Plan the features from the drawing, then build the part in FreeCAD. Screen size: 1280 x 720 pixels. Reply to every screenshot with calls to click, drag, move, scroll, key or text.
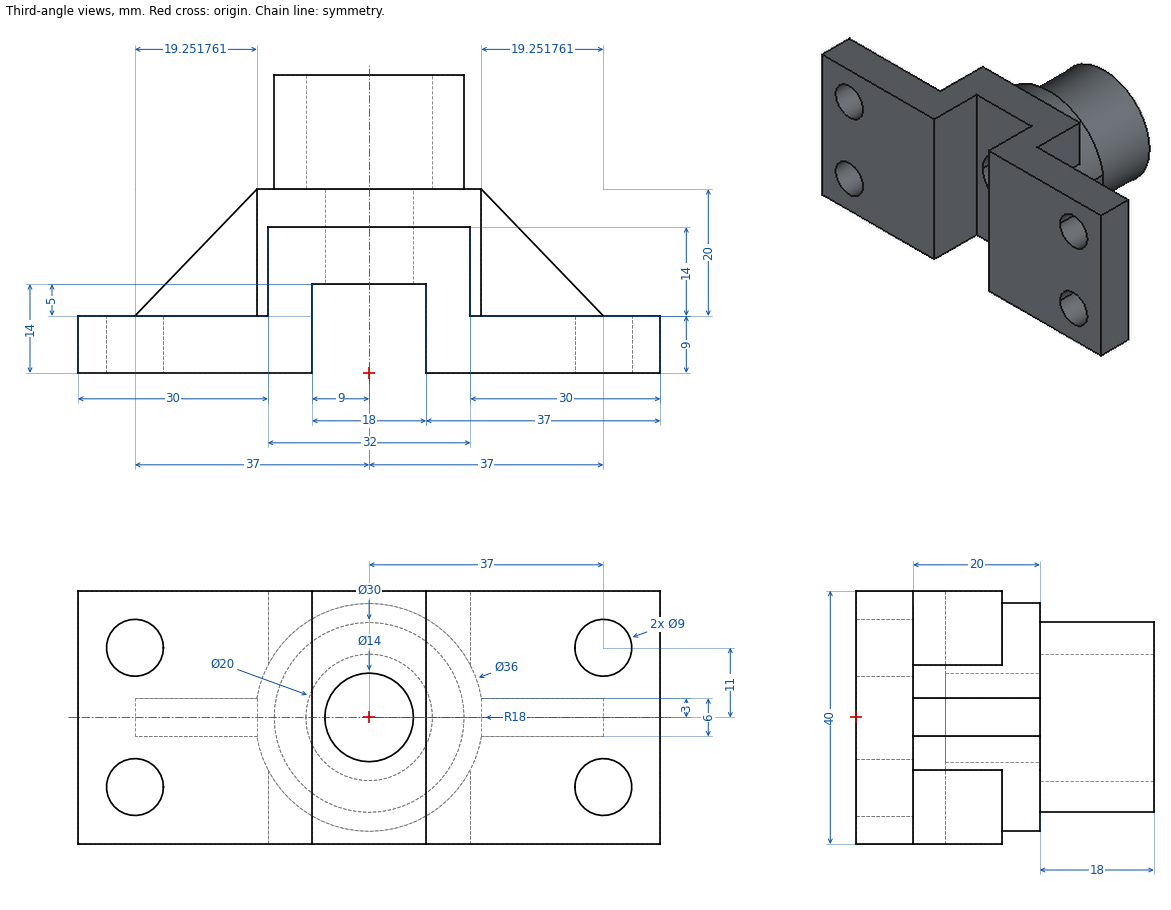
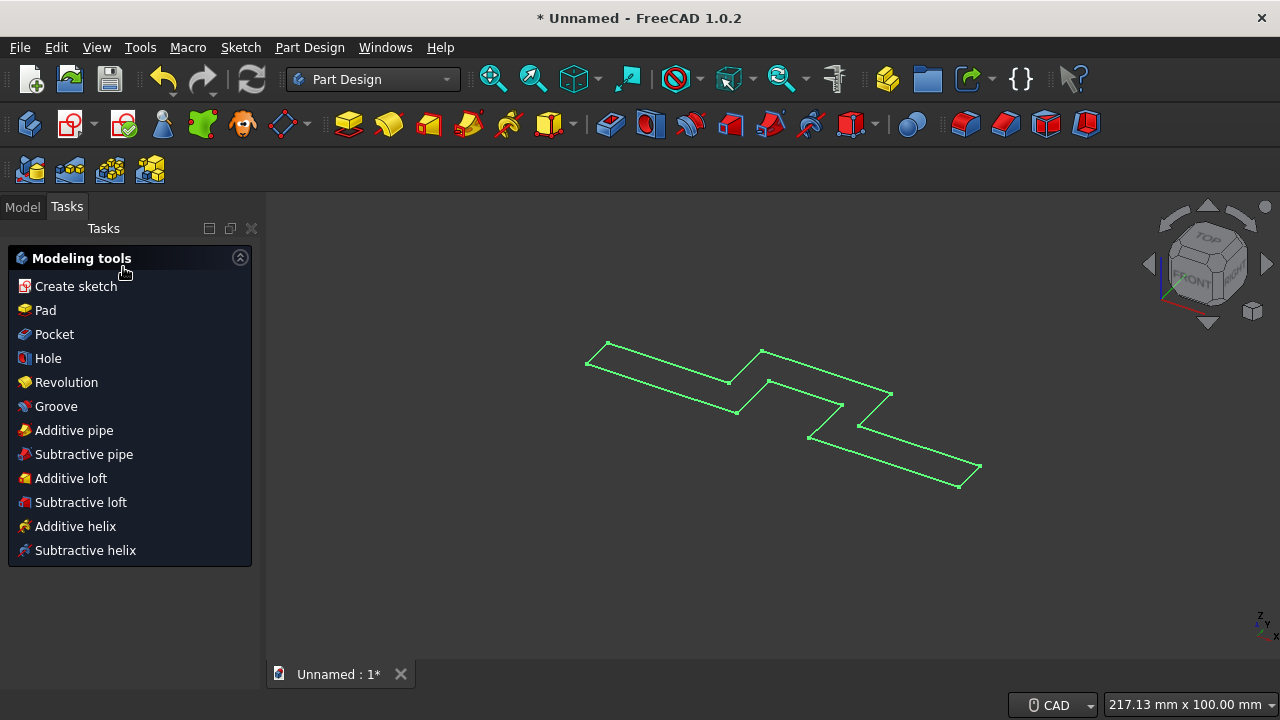
click(350, 124)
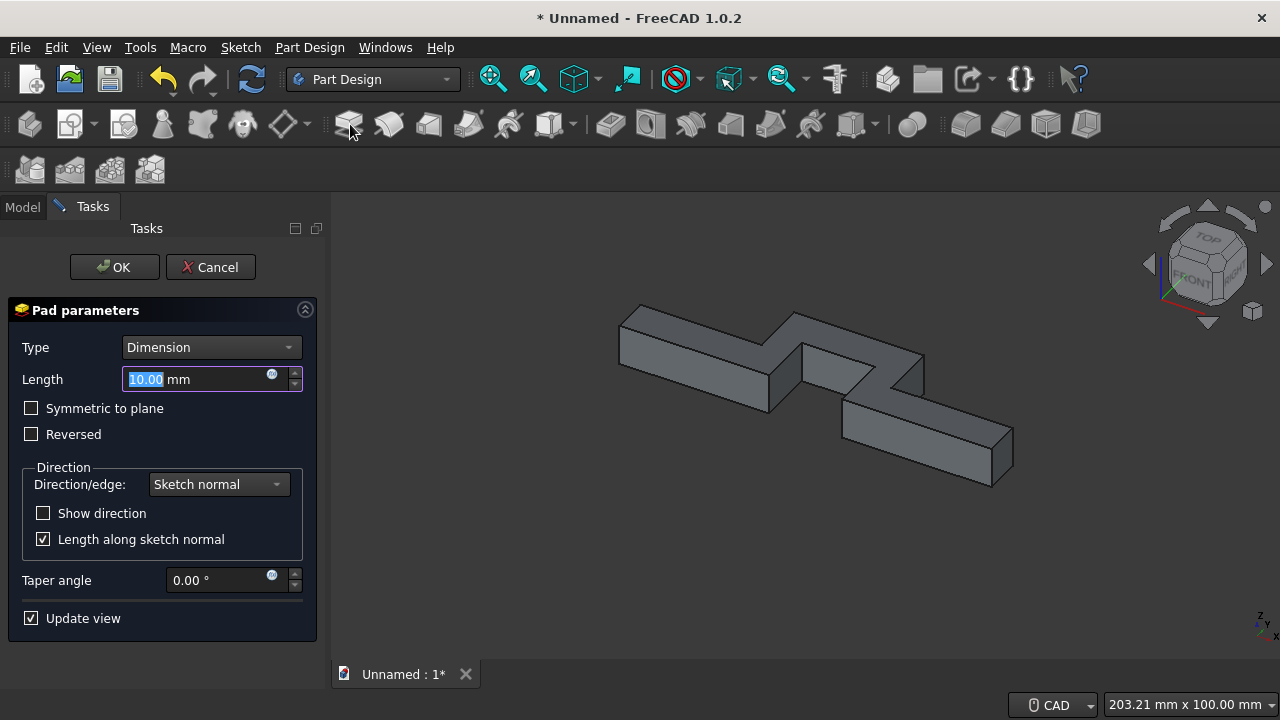
text(40)
key(Tab)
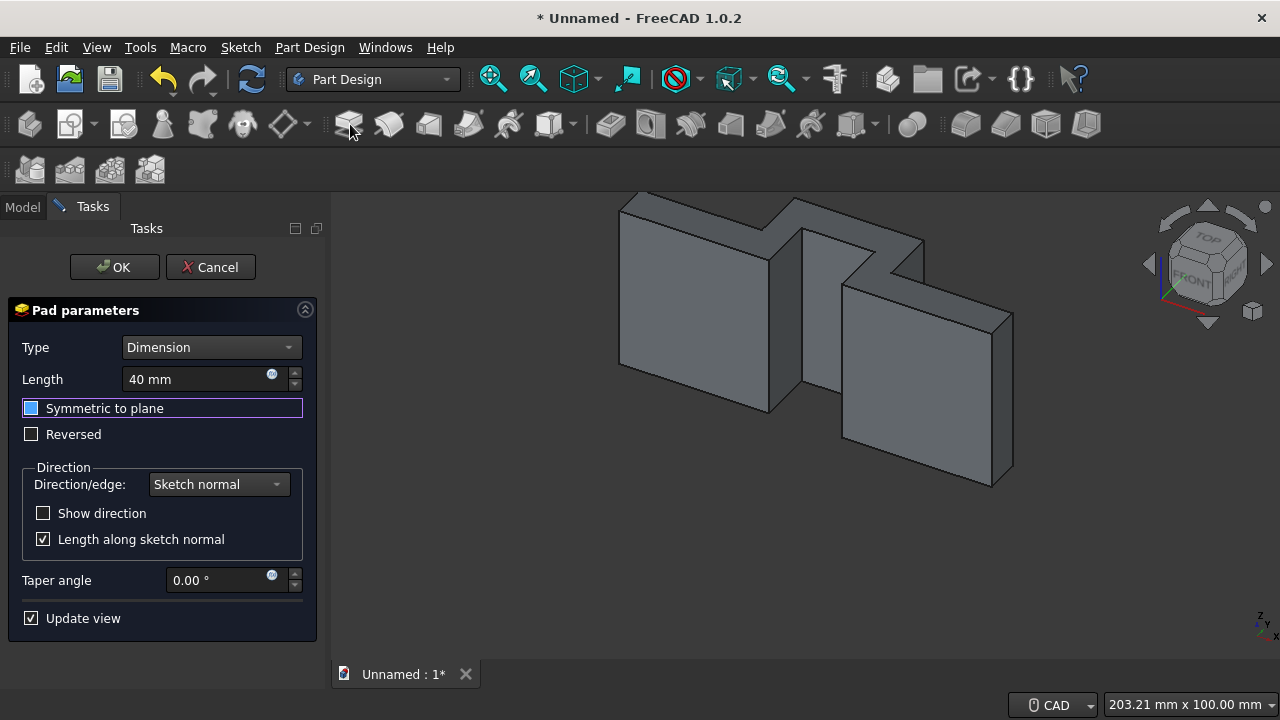
click(30, 408)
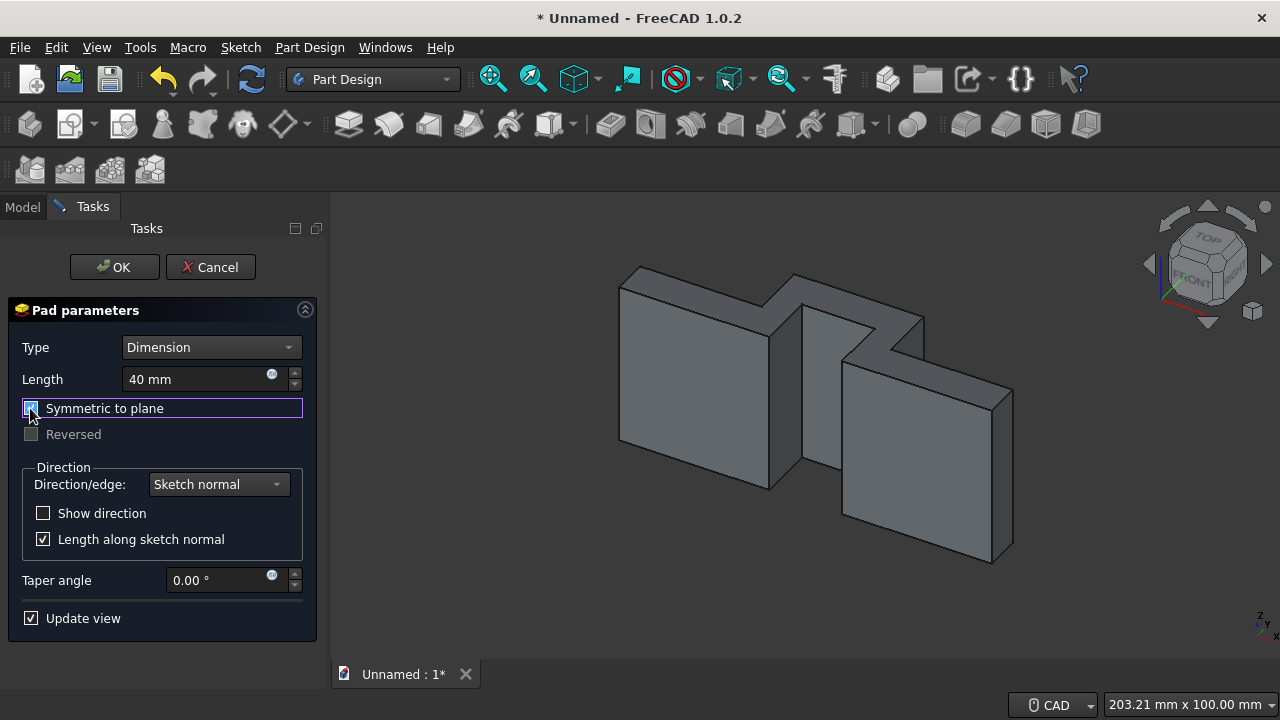
click(115, 267)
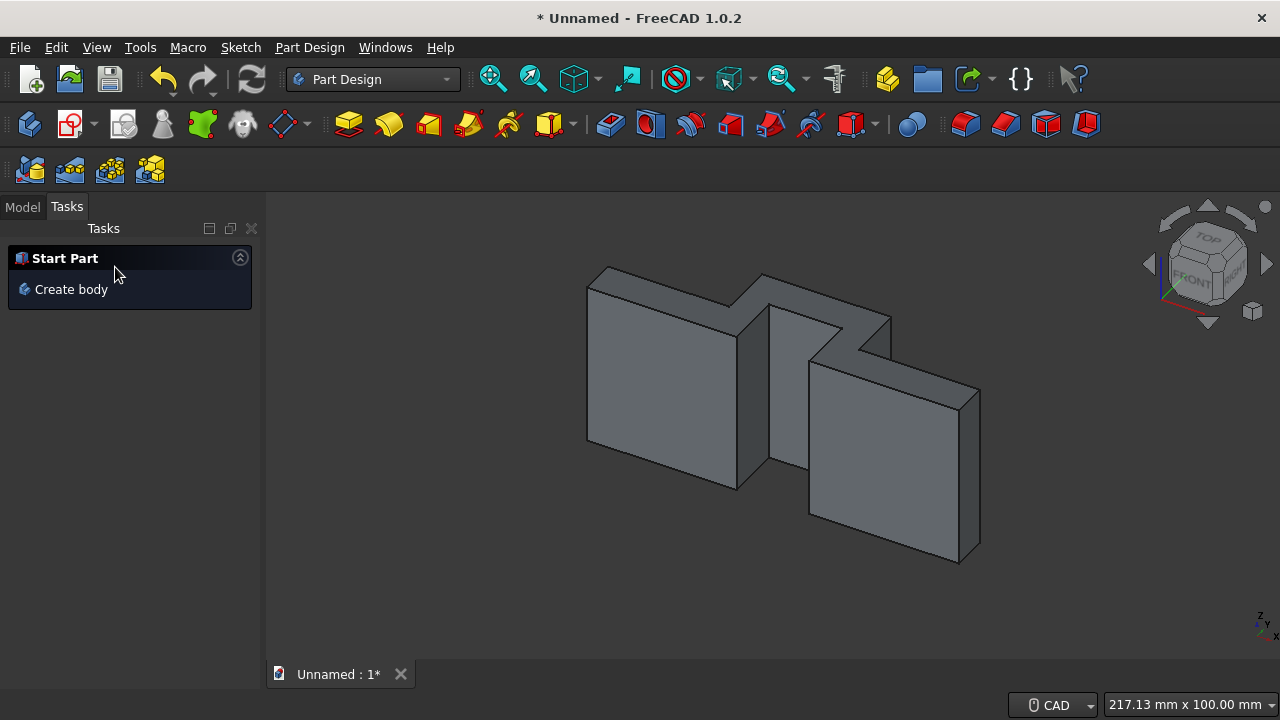
key(4)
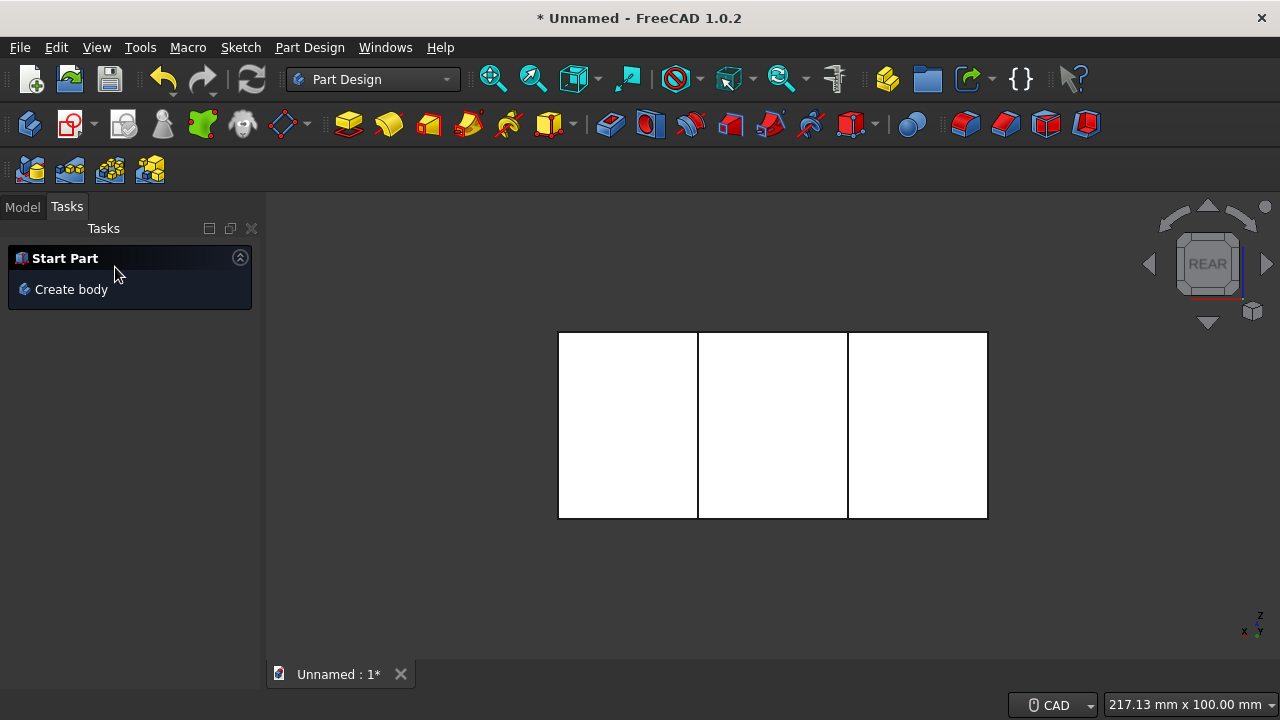
key(v)
key(f)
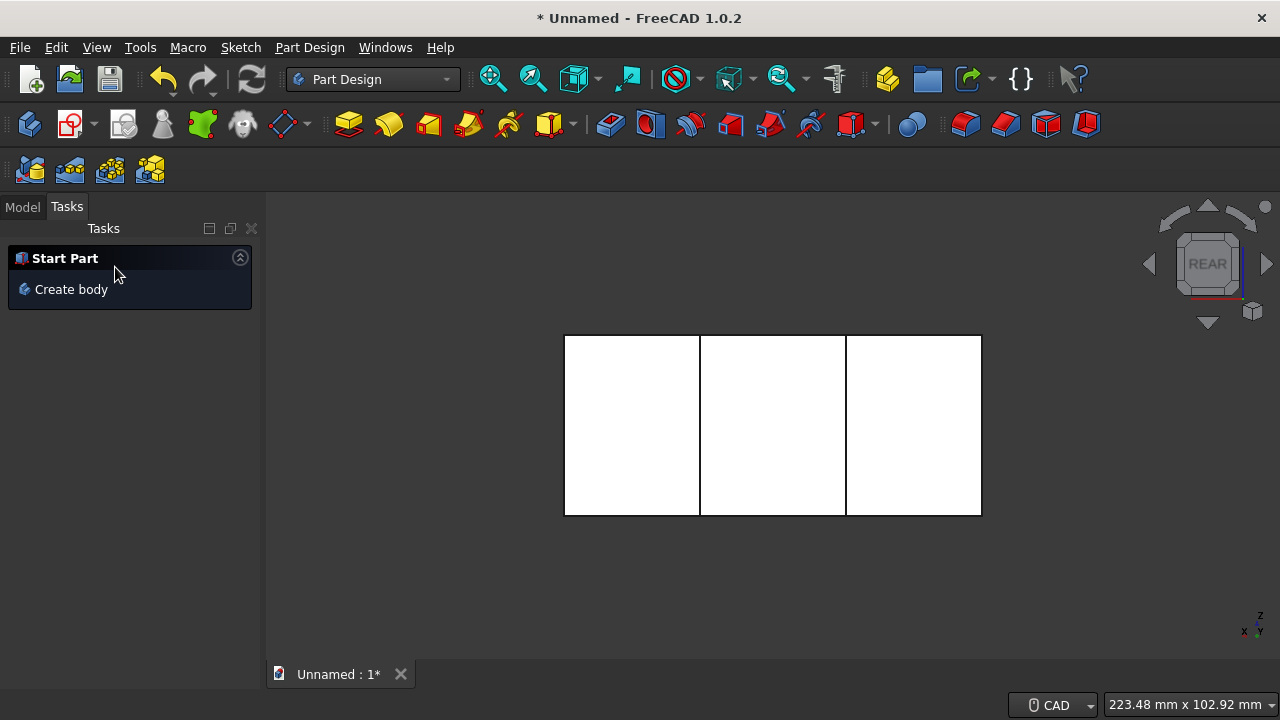
click(632, 425)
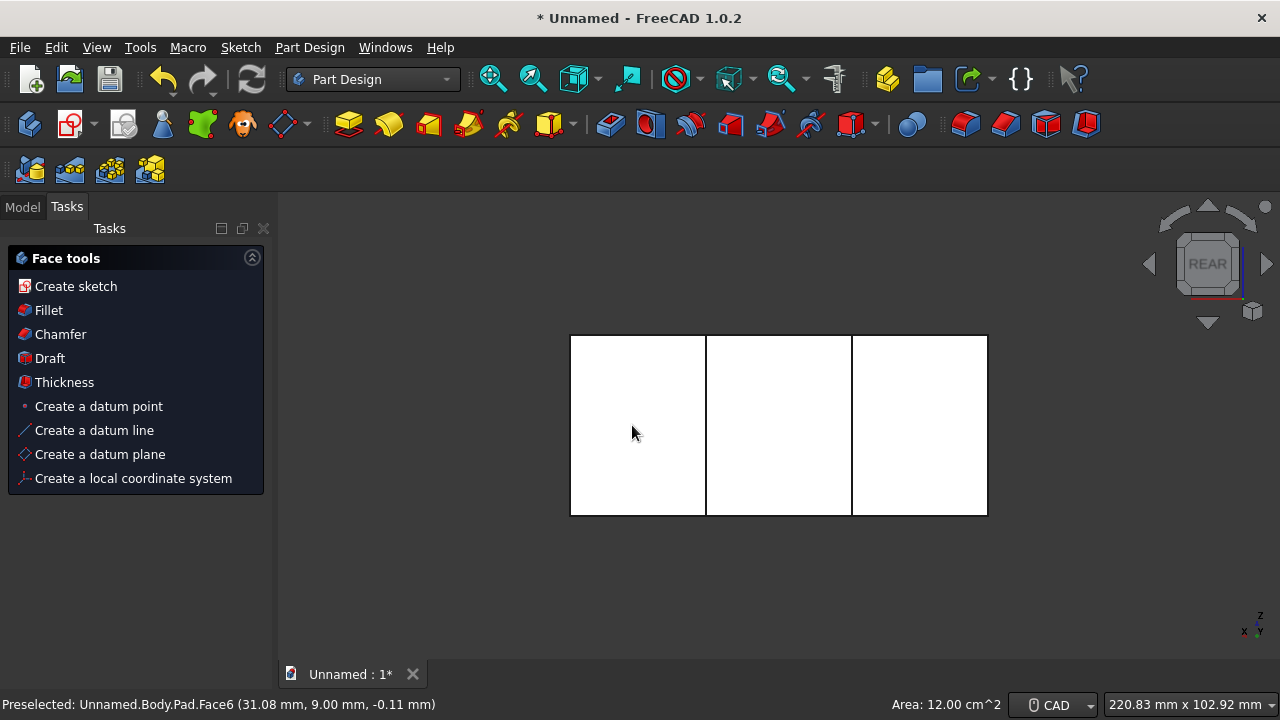
click(70, 124)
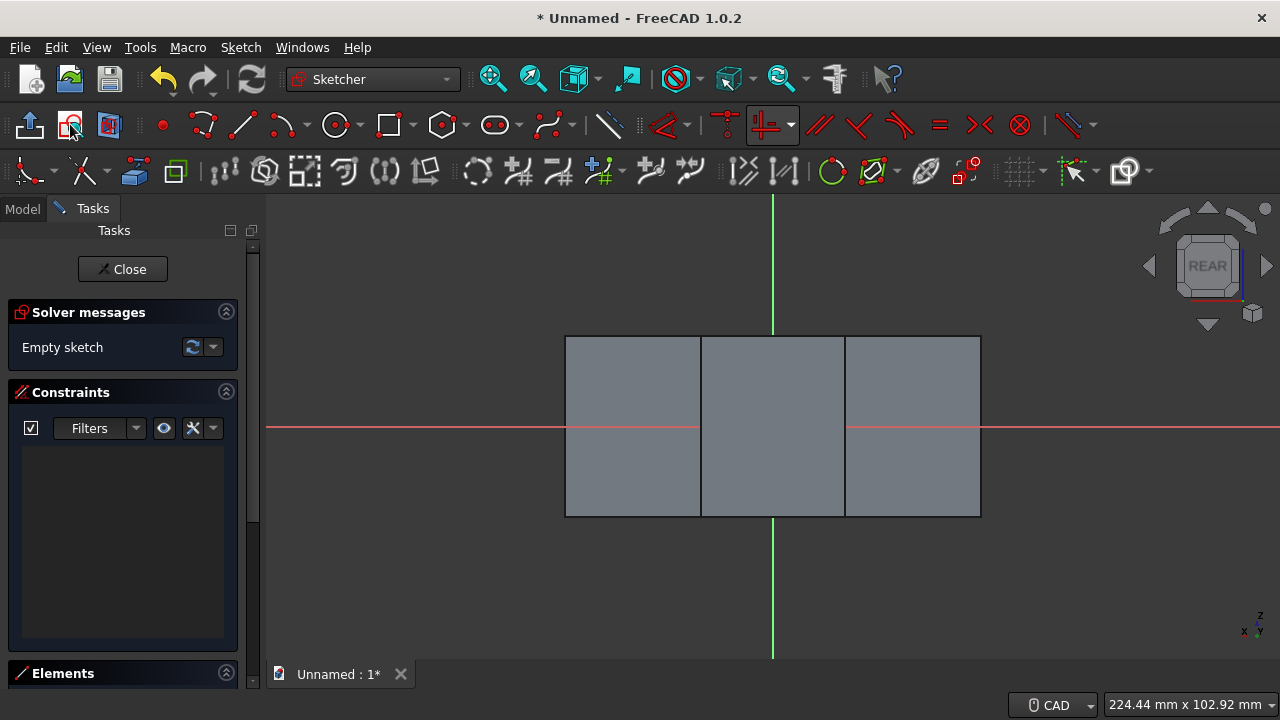
scroll(856, 427, up, 3)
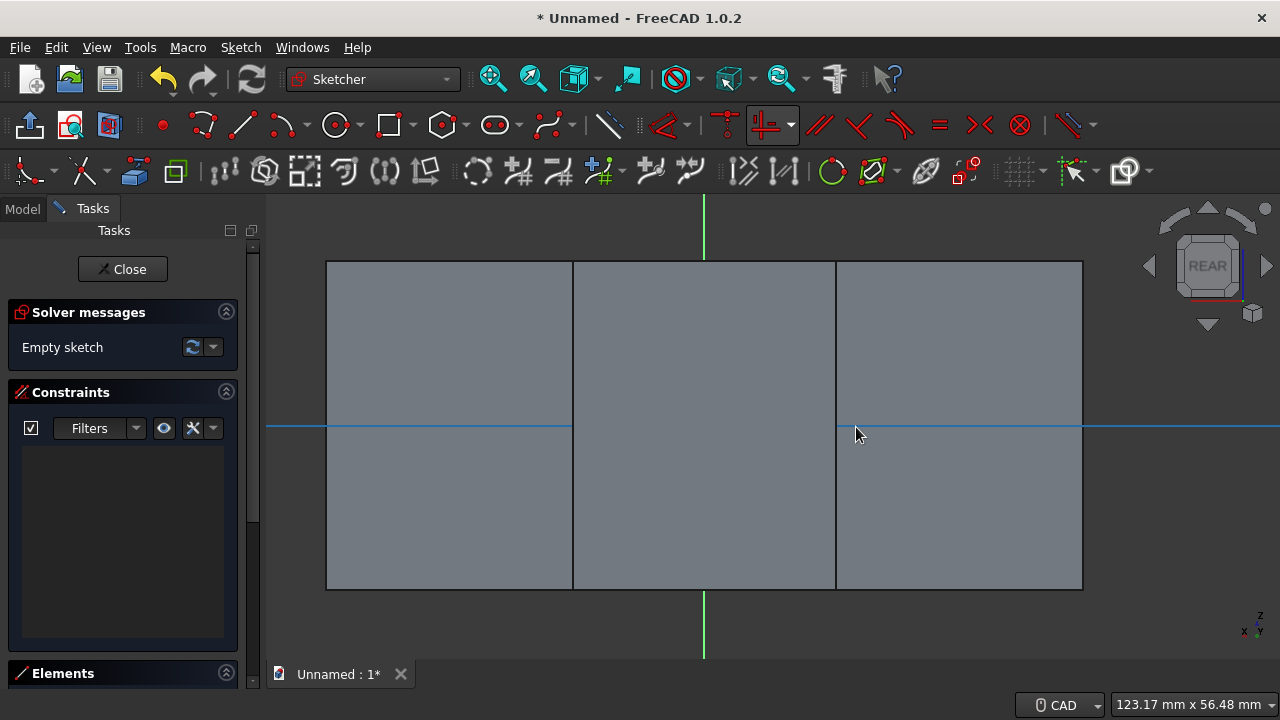
key(g)
key(c)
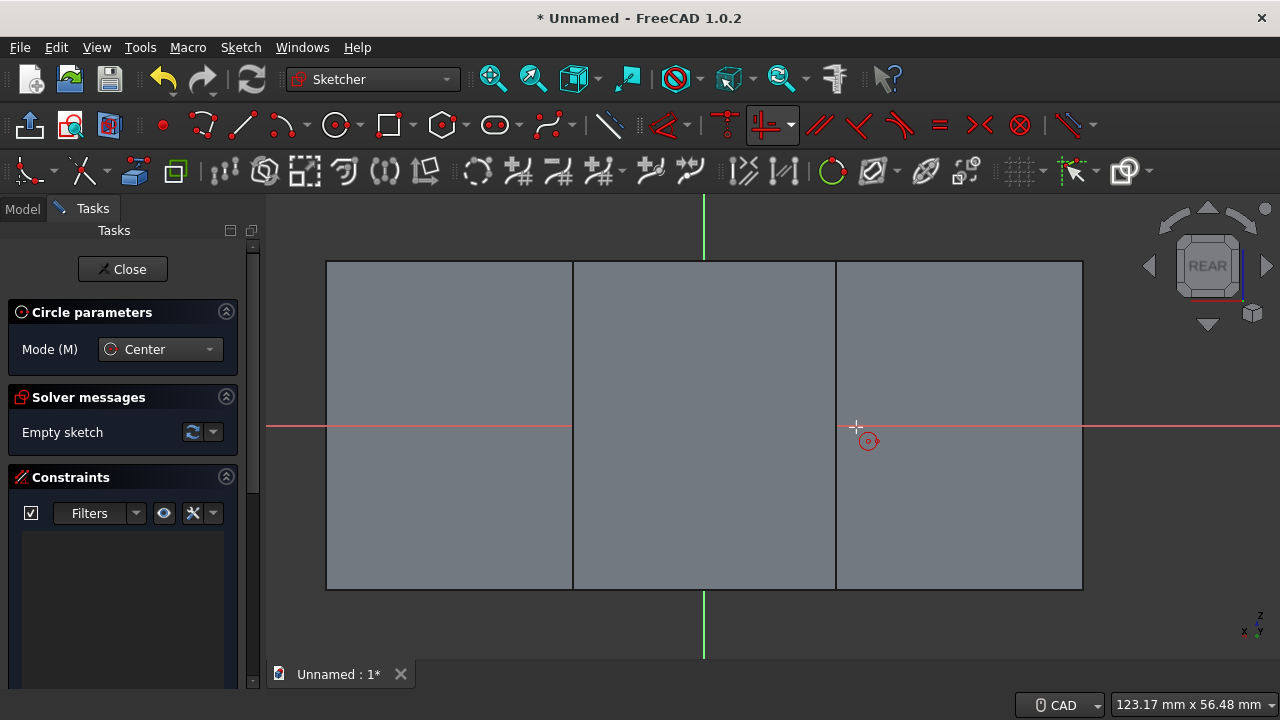
click(704, 426)
click(809, 321)
key(Escape)